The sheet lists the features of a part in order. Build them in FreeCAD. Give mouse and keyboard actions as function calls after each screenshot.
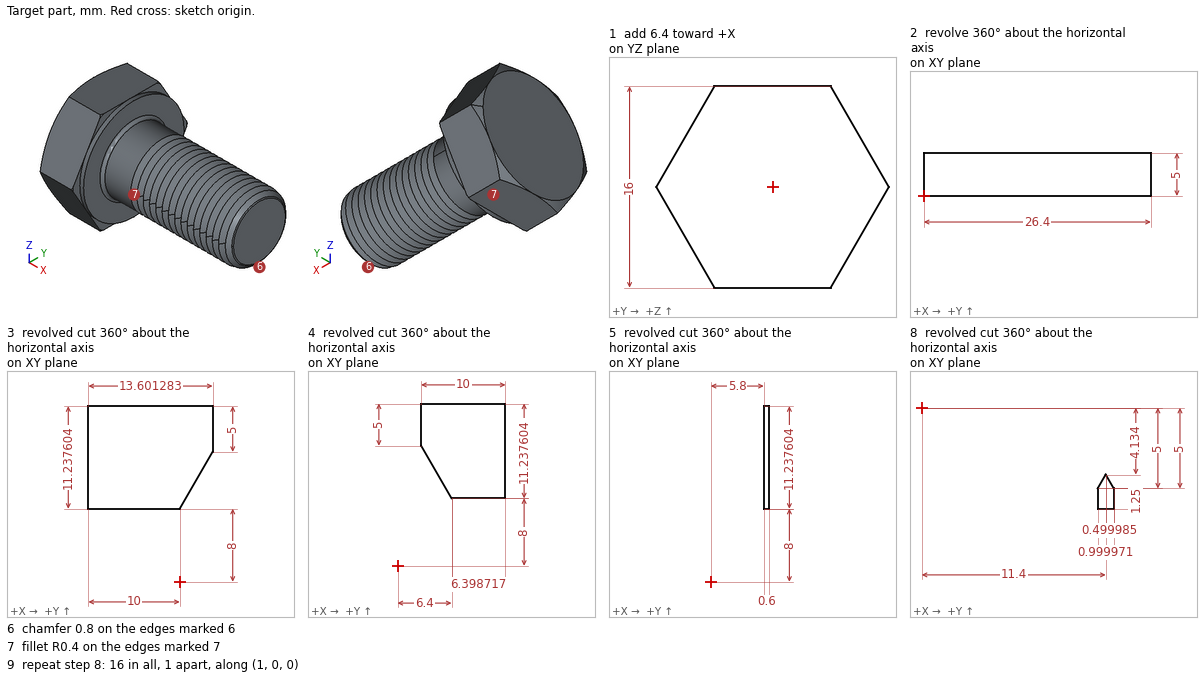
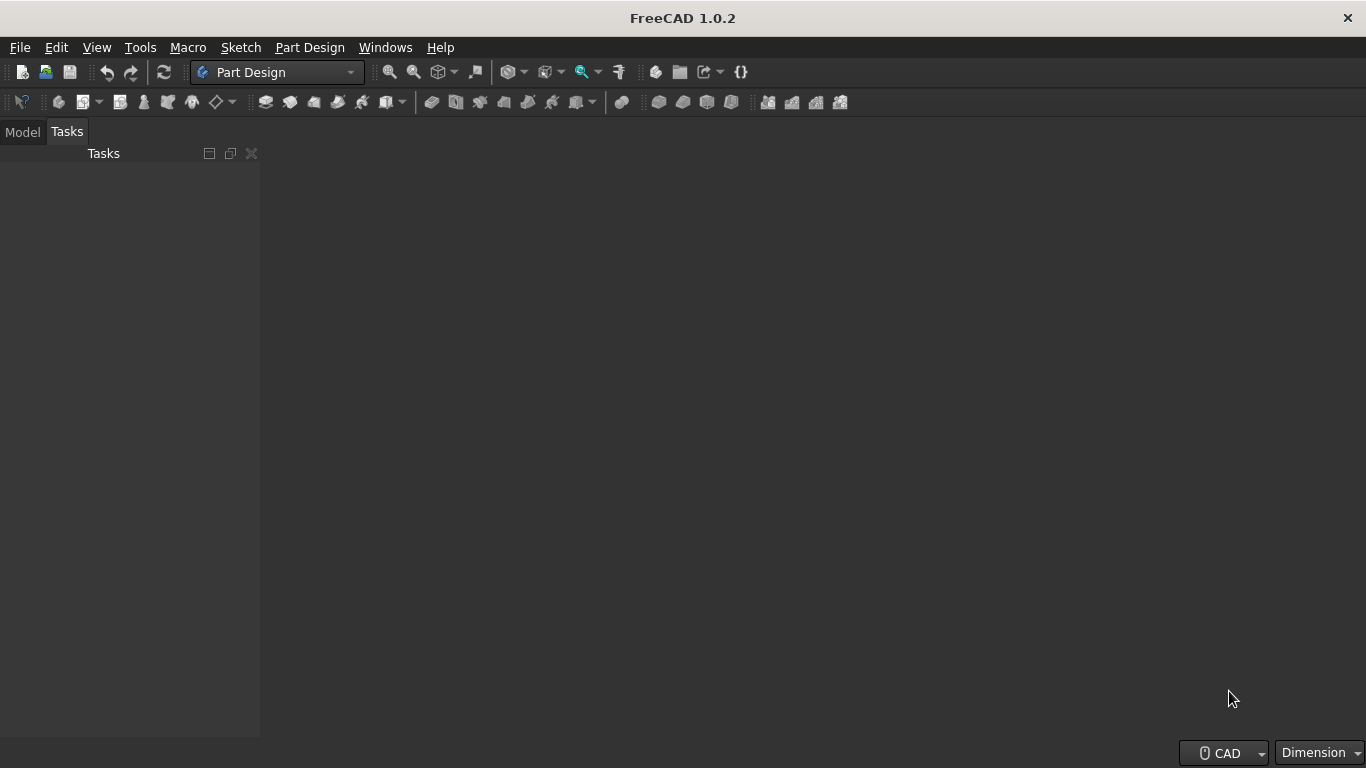
click(22, 72)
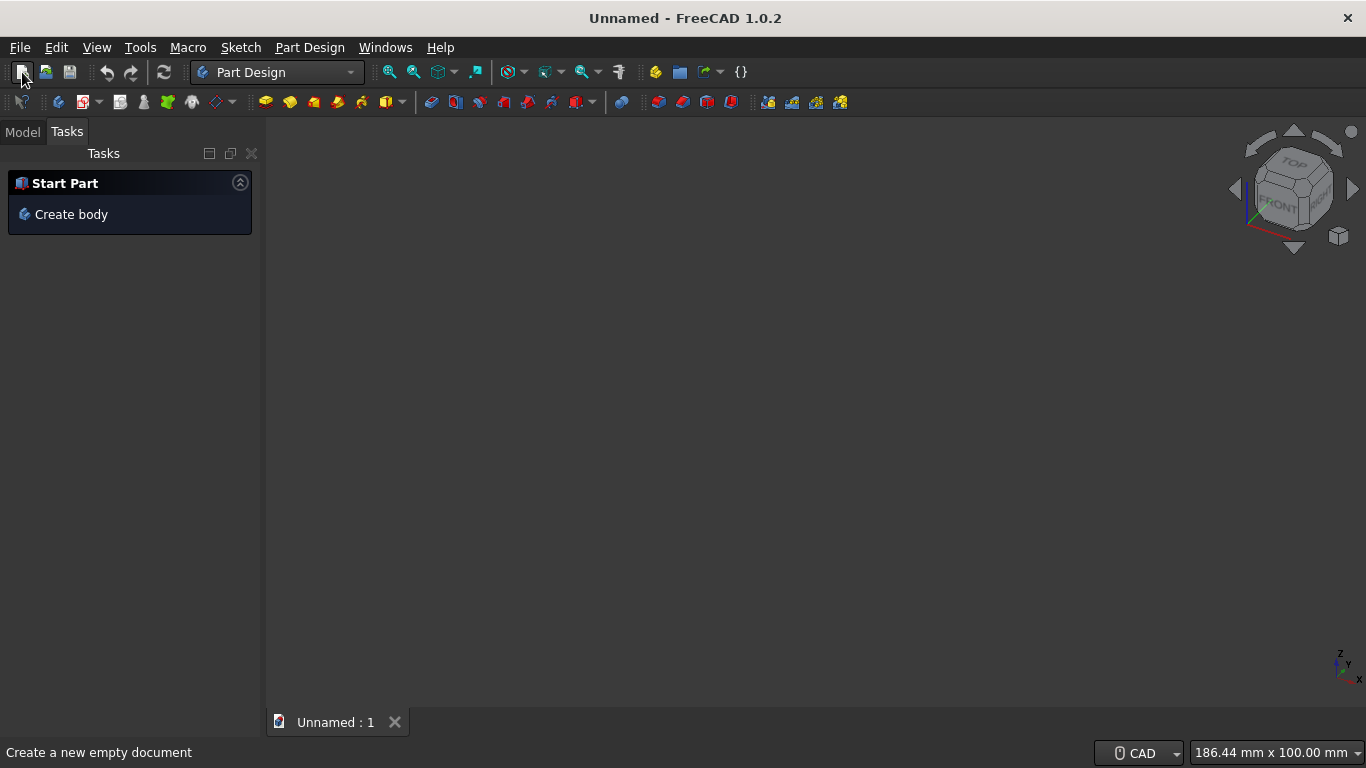
click(84, 102)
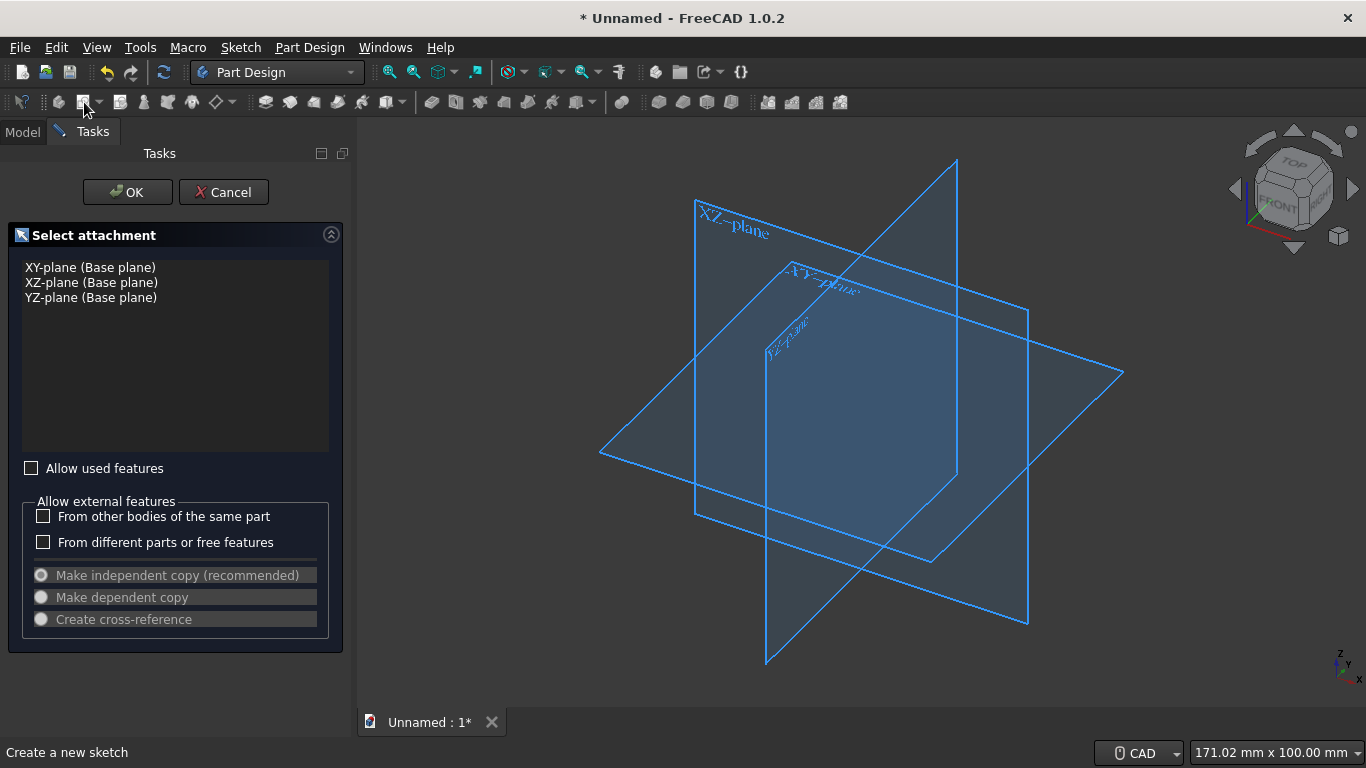
click(82, 298)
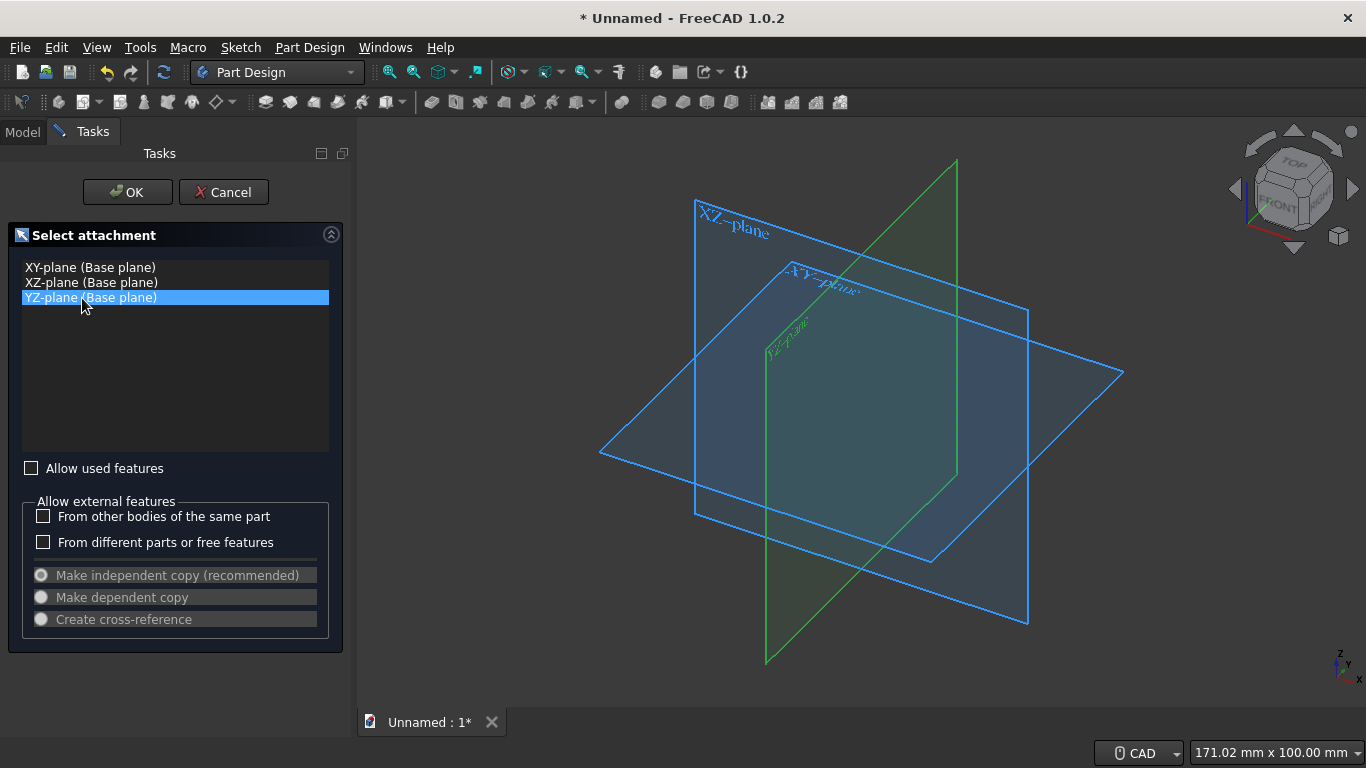
click(128, 192)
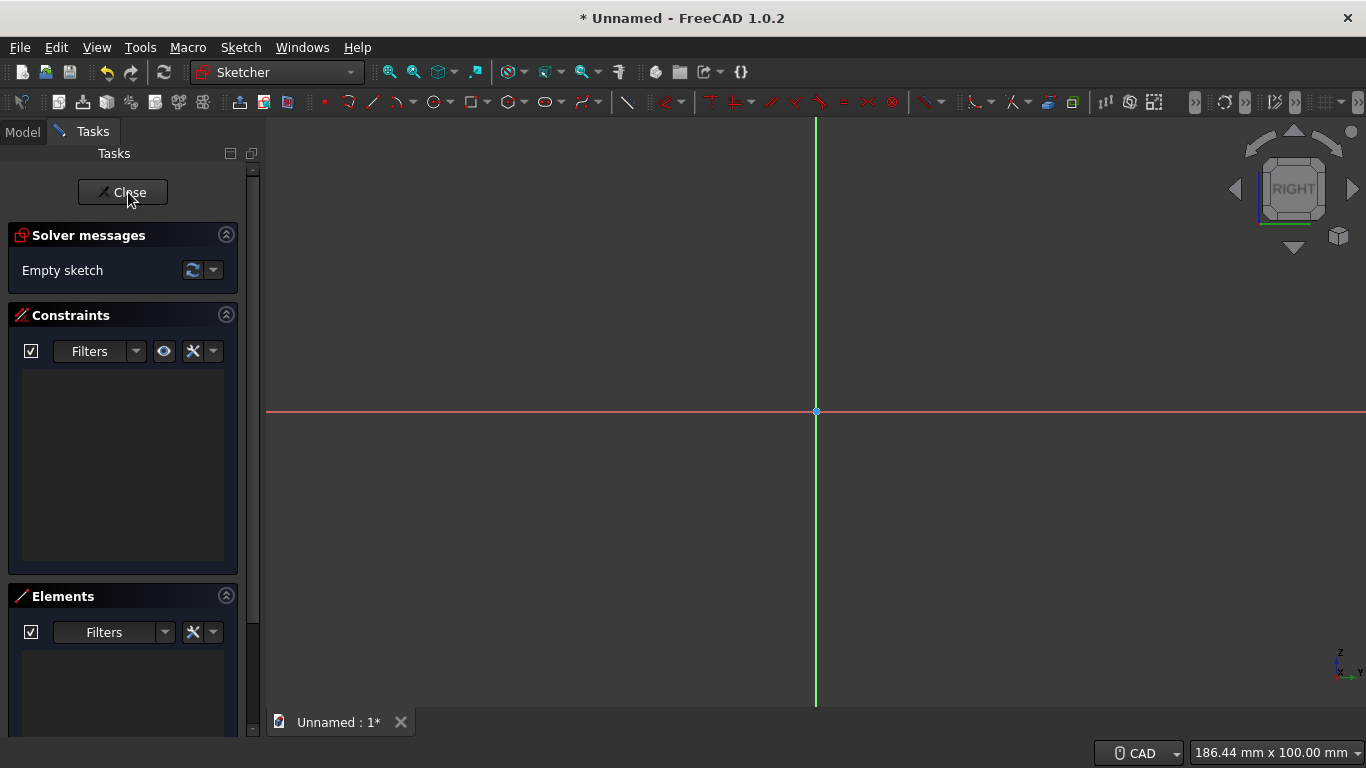
scroll(838, 412, up, 7)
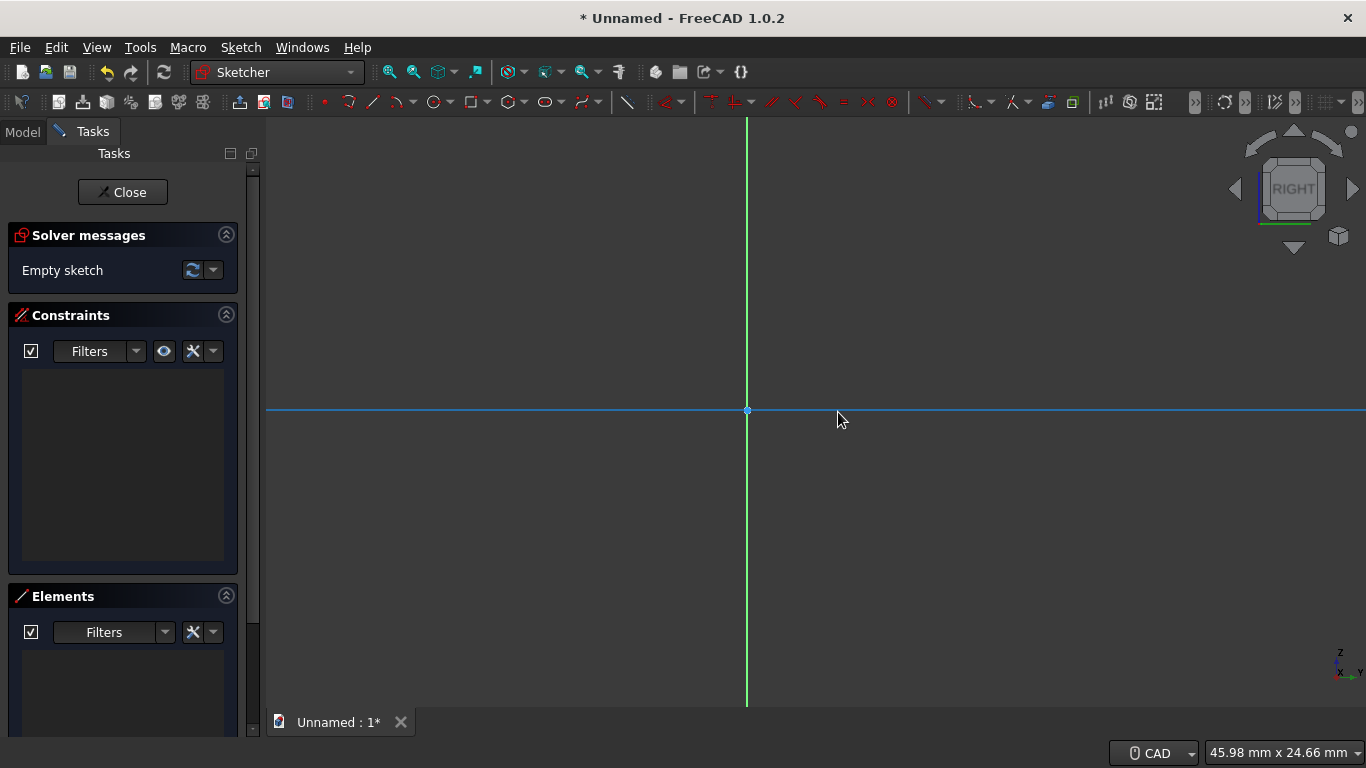
click(508, 102)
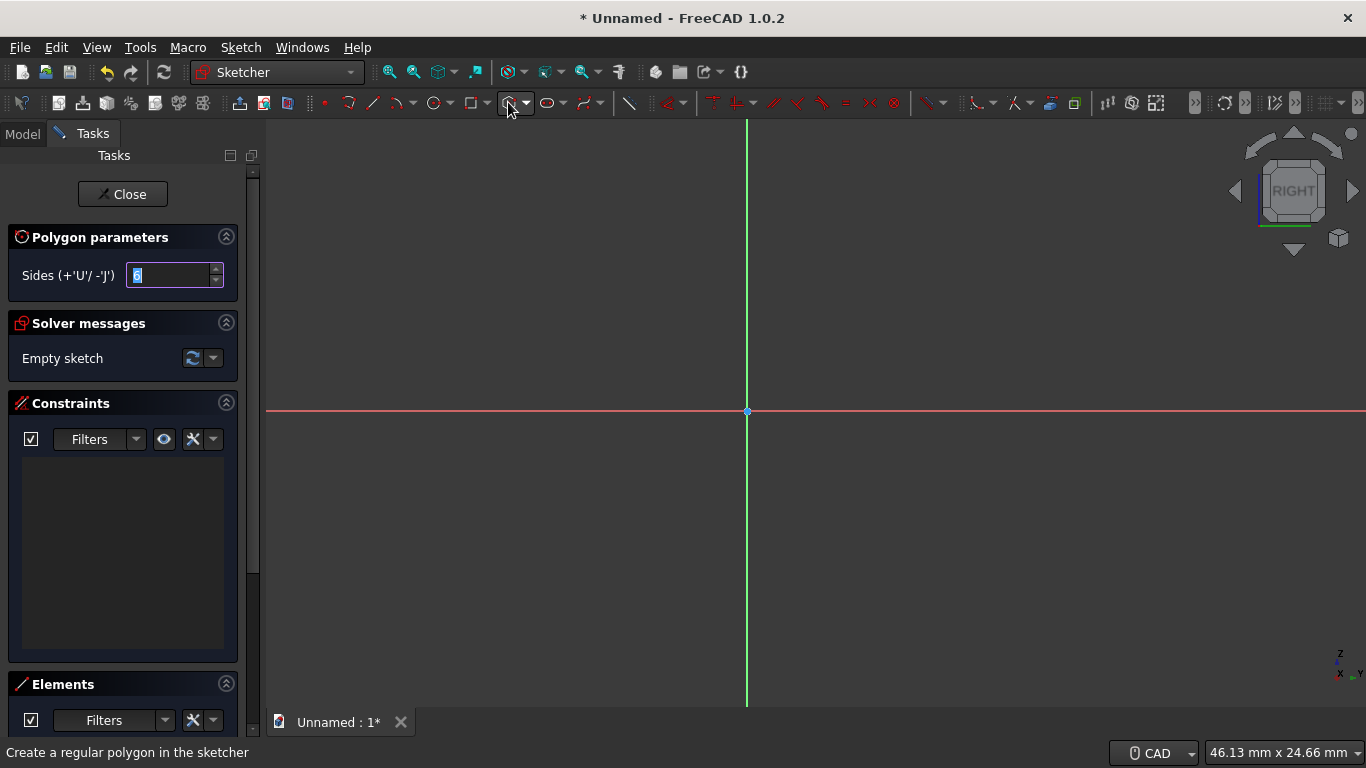
click(747, 411)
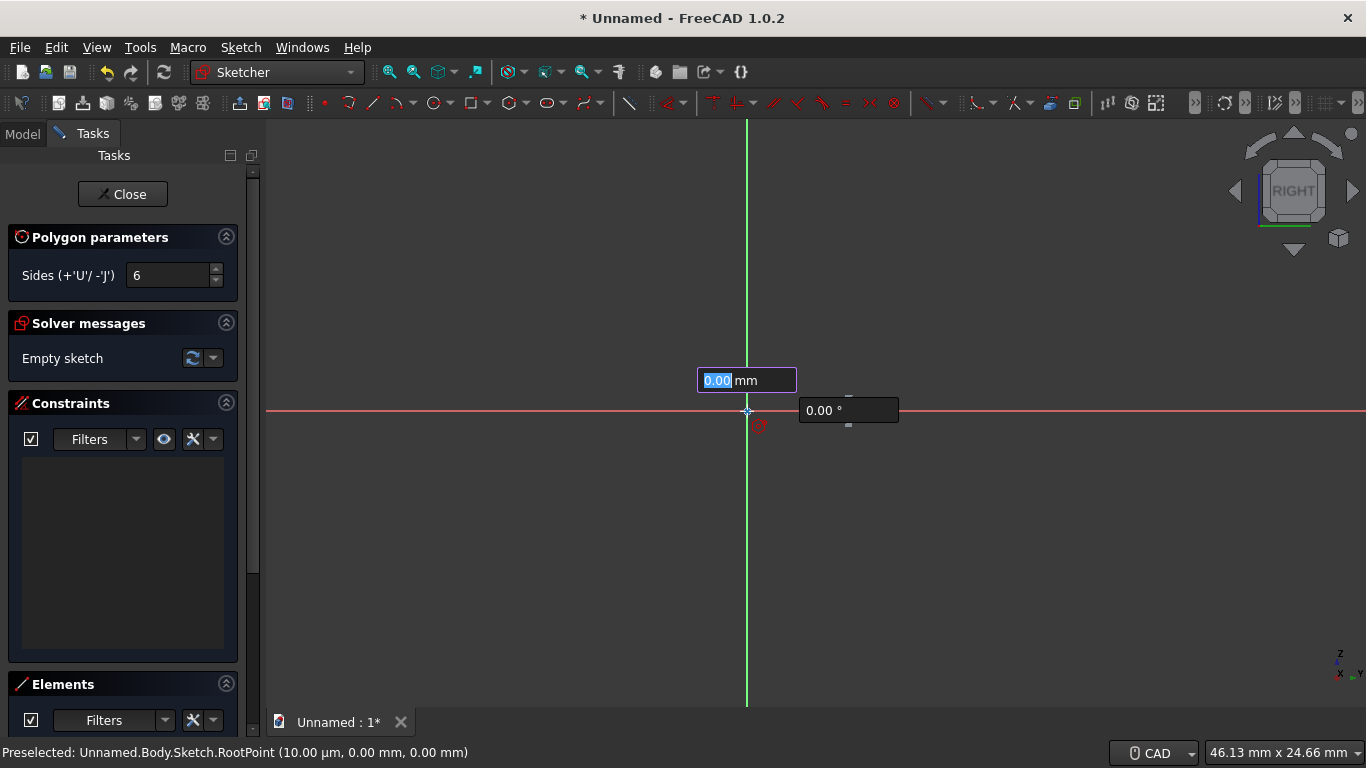
click(968, 411)
right_click(968, 411)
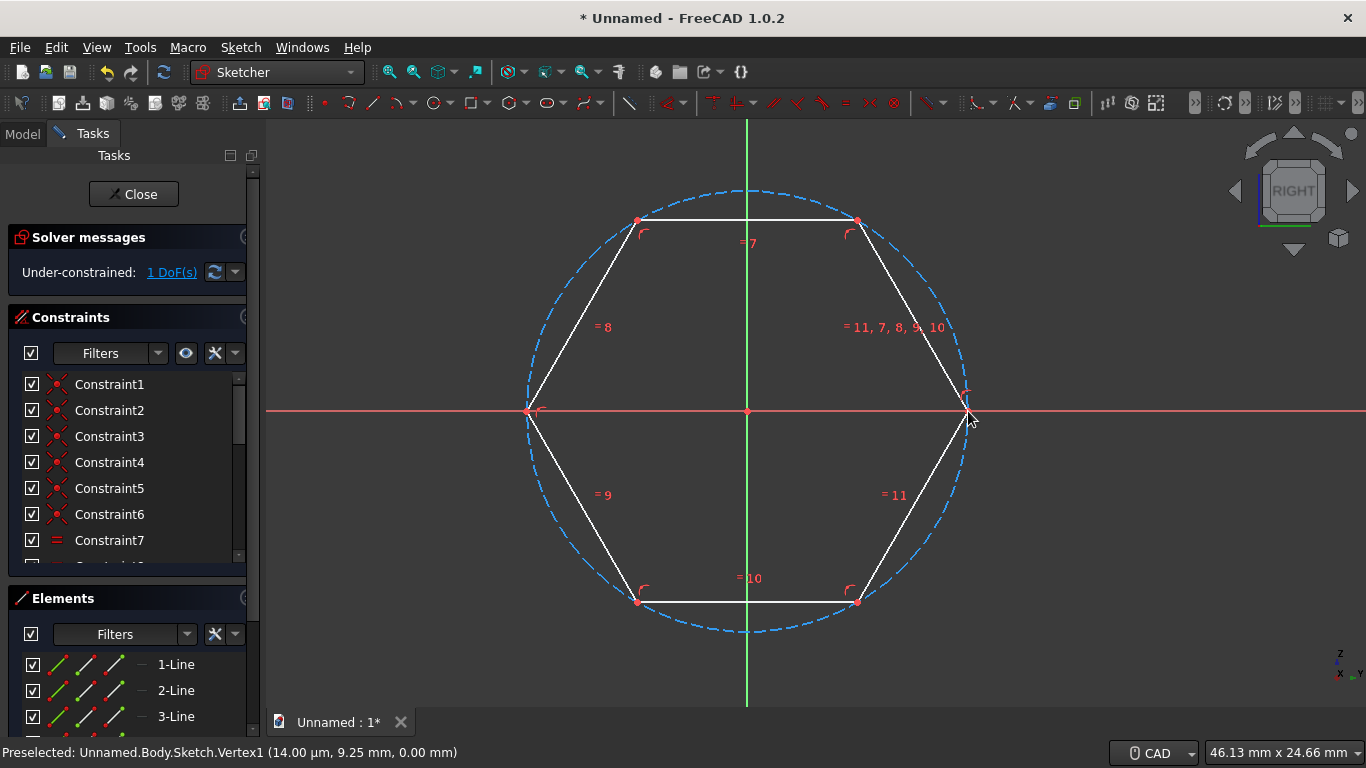
key(d)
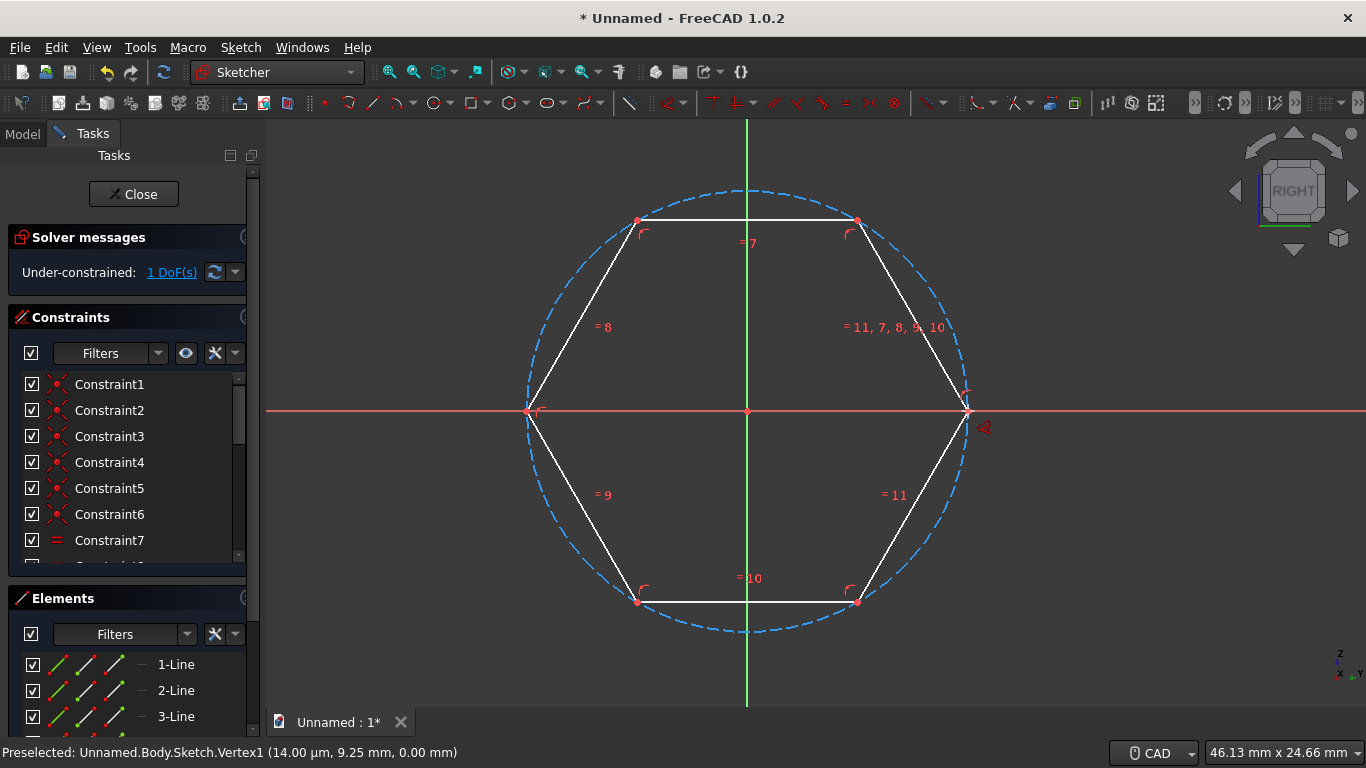
click(637, 602)